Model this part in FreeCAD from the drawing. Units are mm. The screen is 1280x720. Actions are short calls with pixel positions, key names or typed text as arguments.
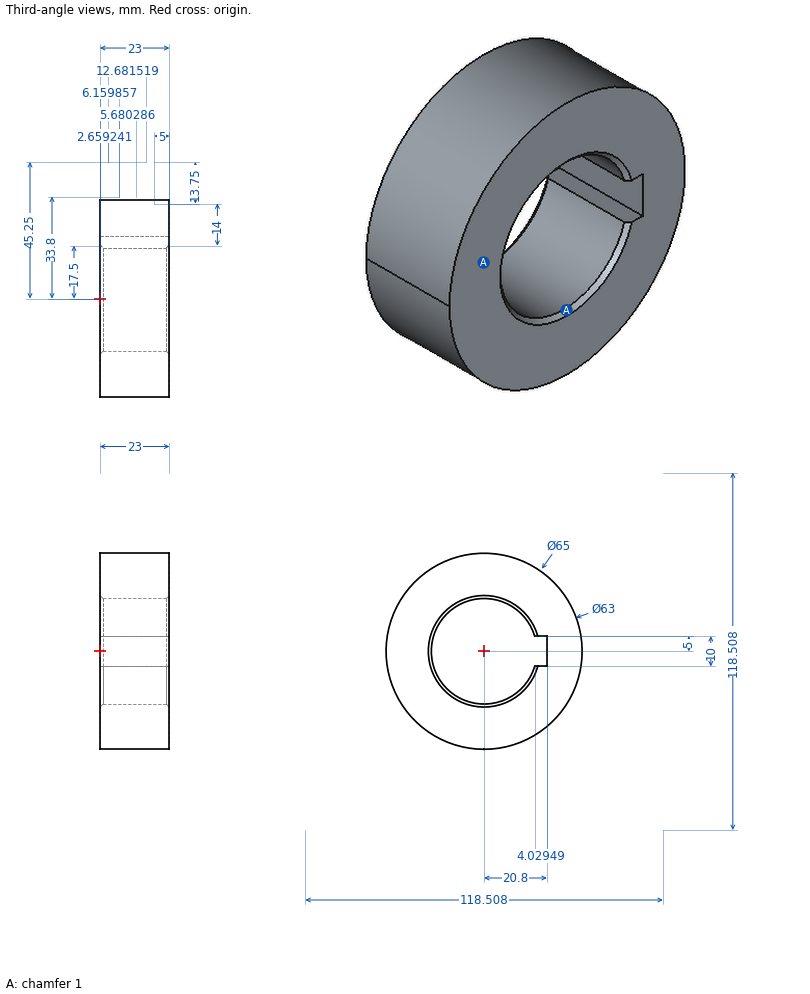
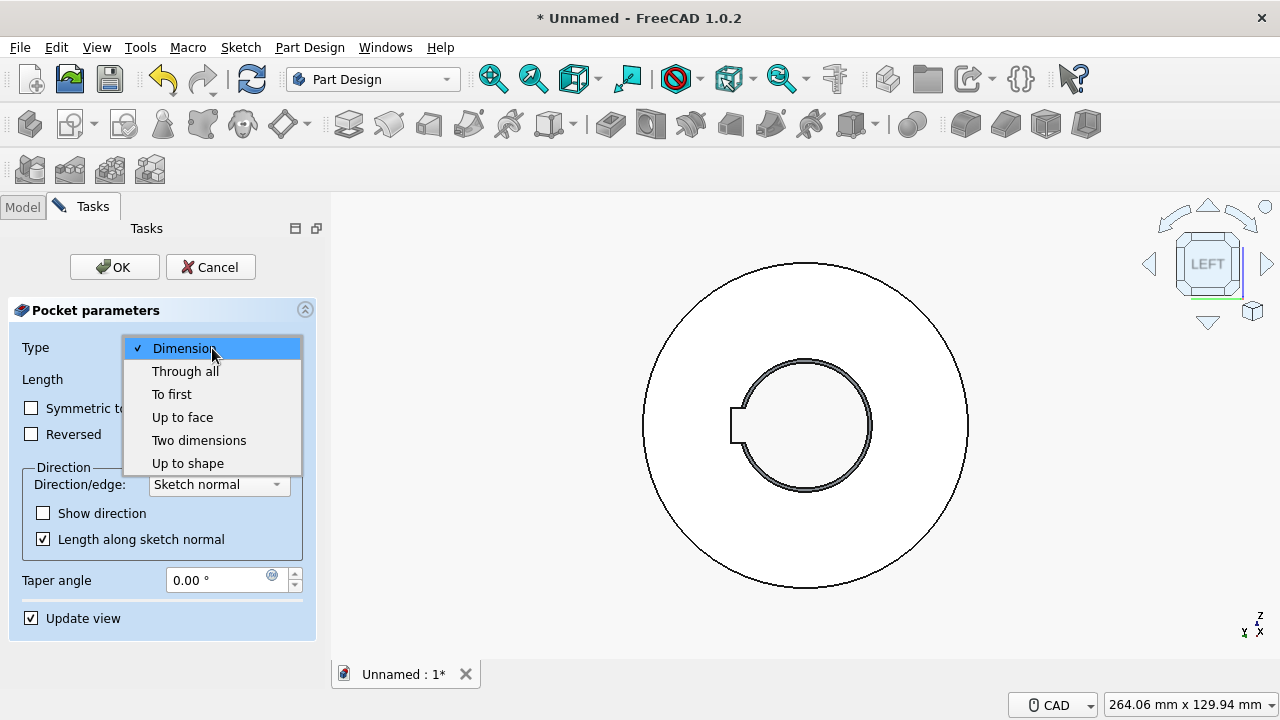
click(212, 440)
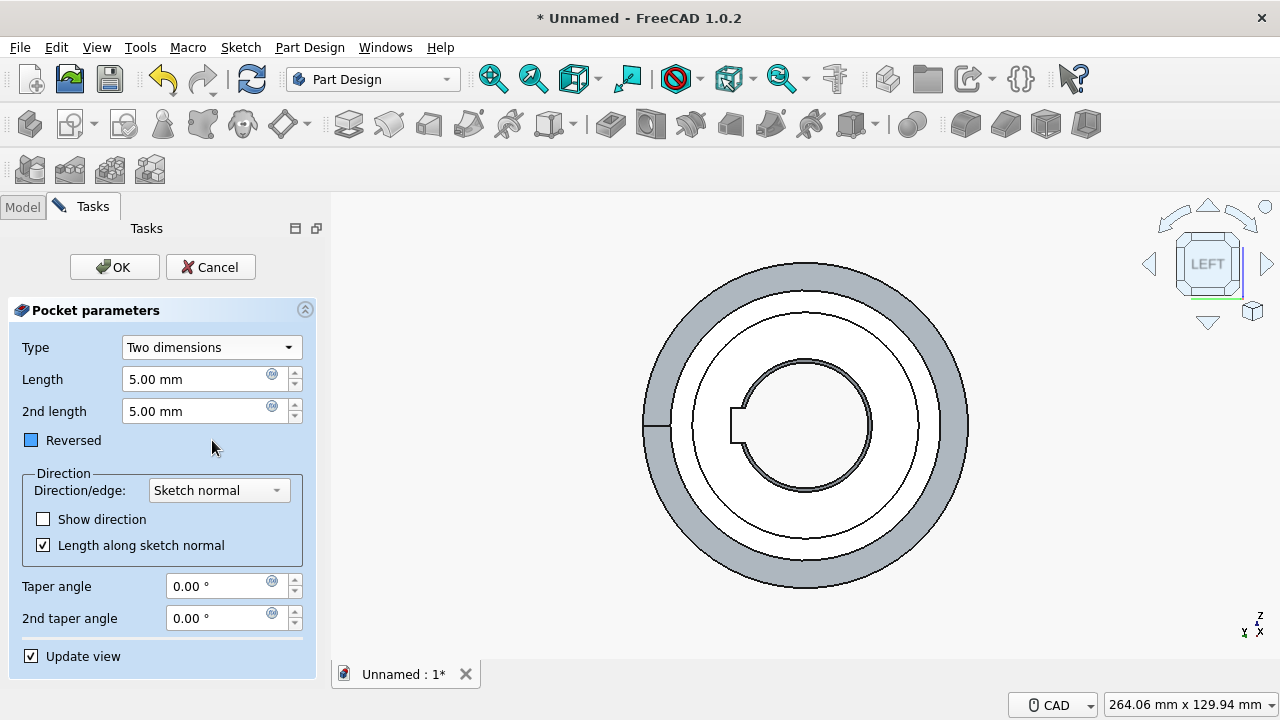
triple_click(204, 379)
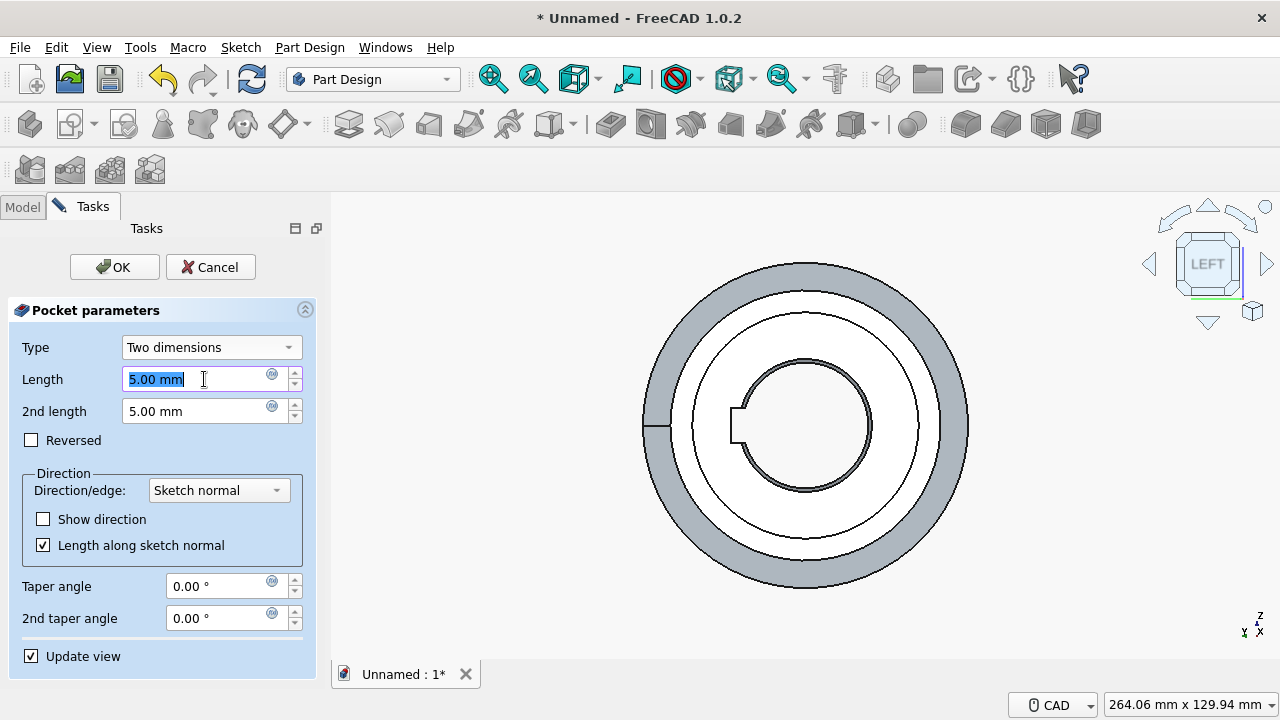
text(23)
key(Tab)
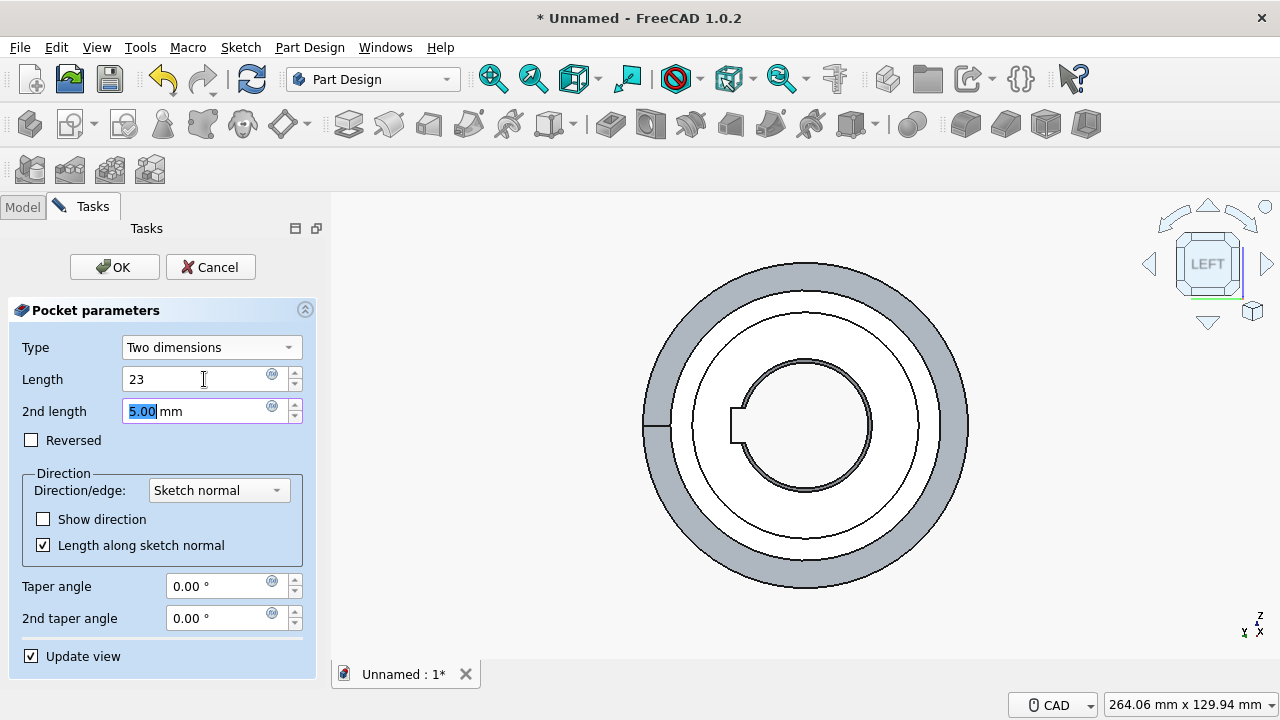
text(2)
key(Tab)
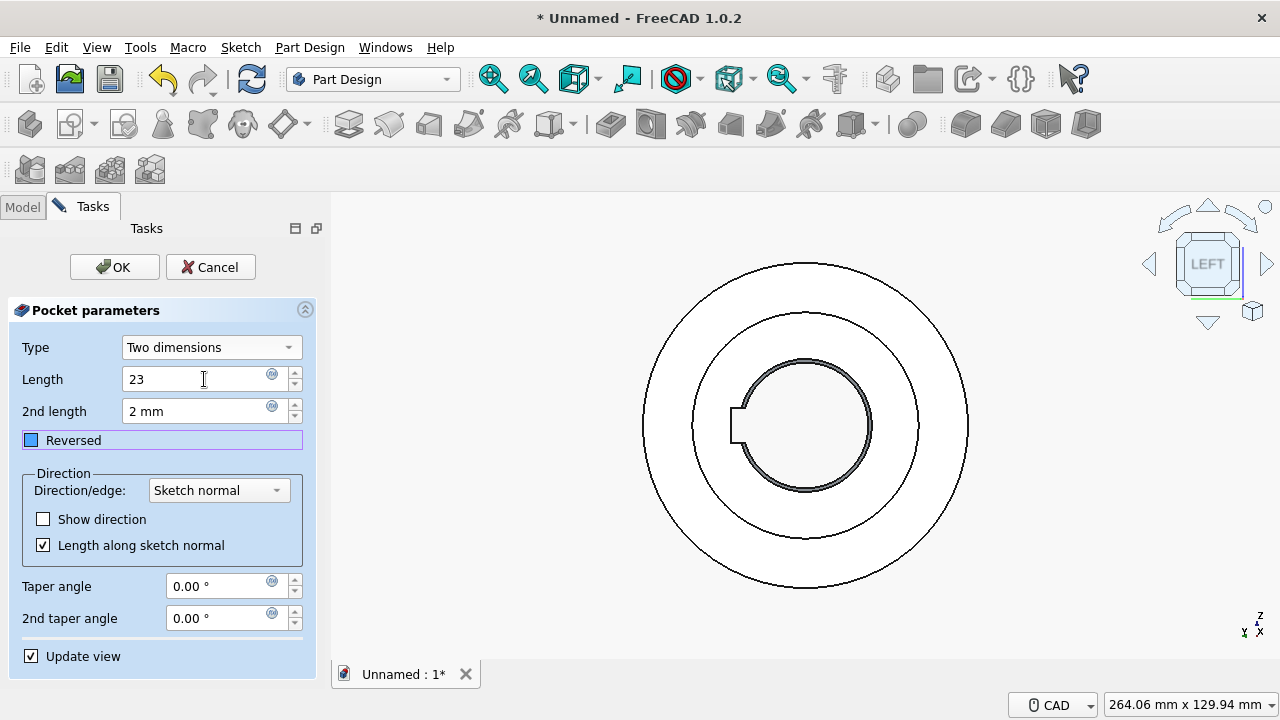
click(30, 440)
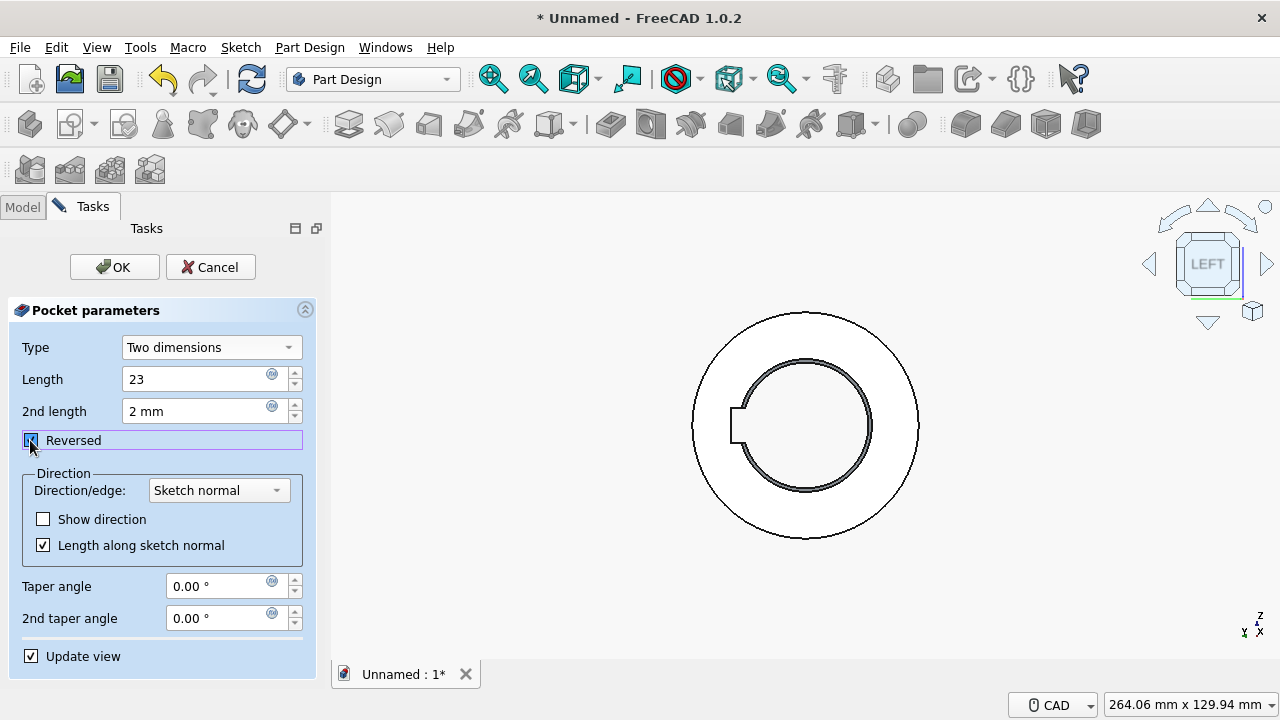
click(115, 267)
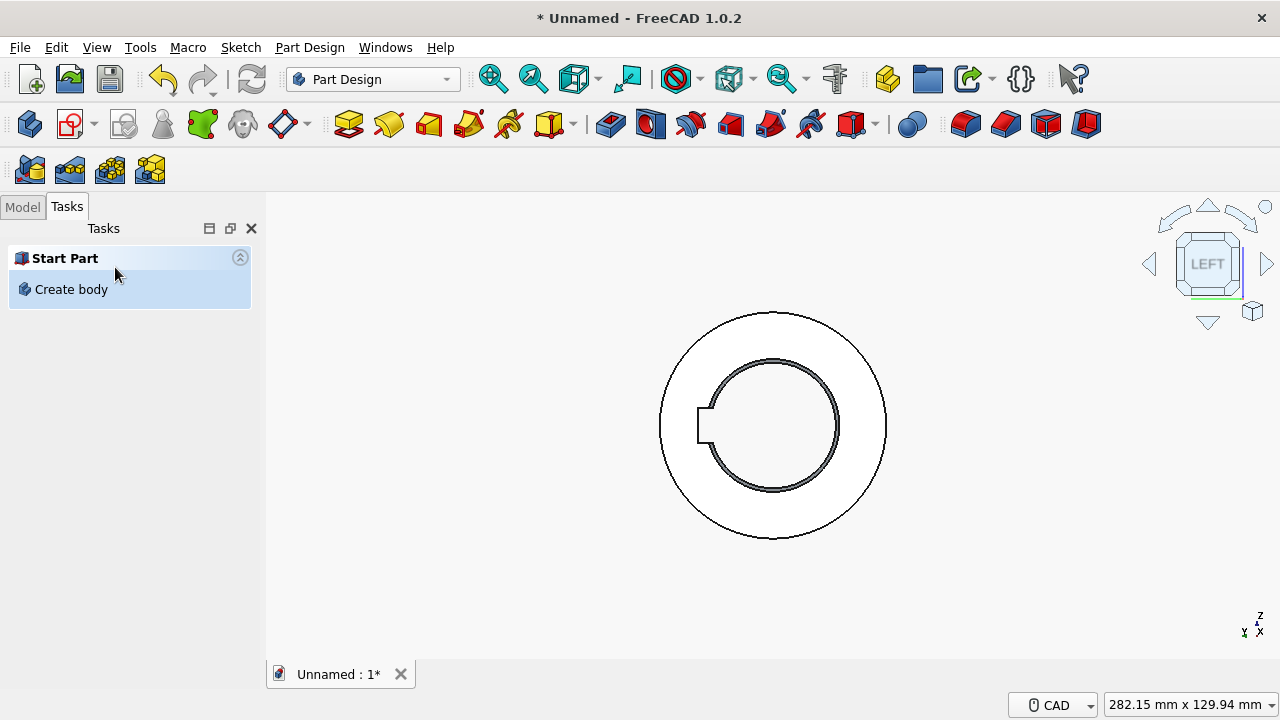
click(838, 489)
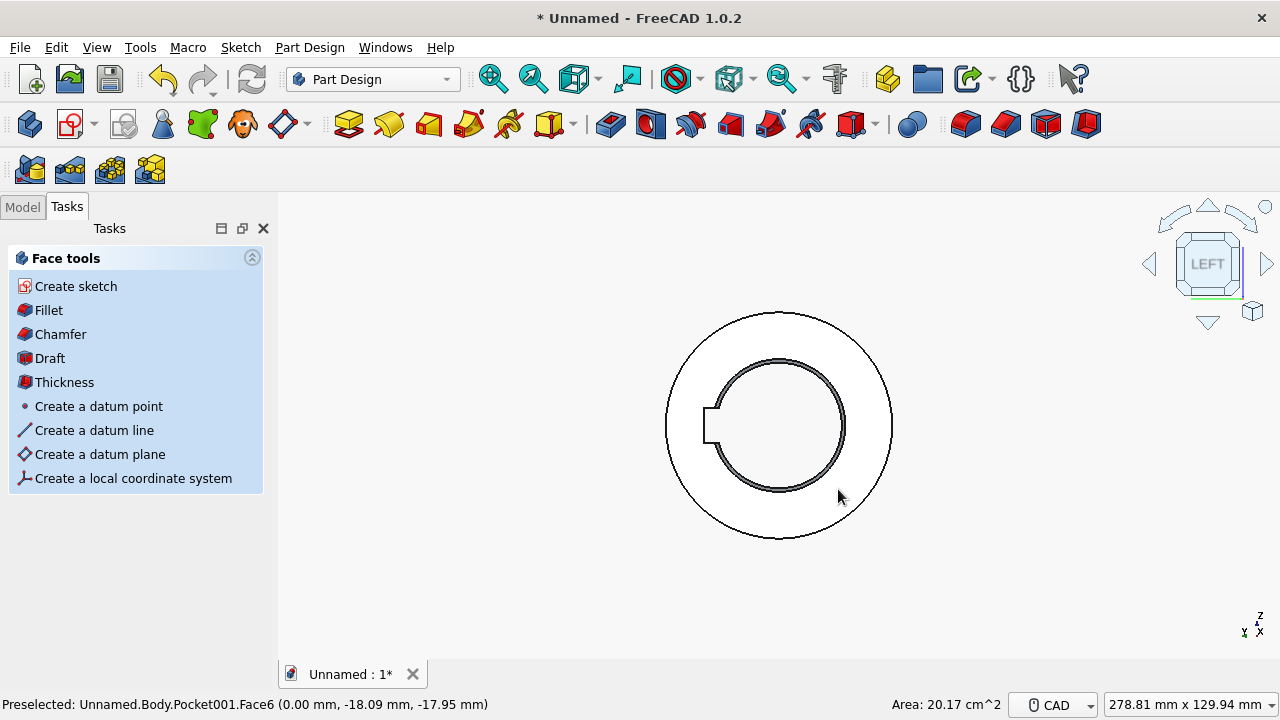
click(70, 124)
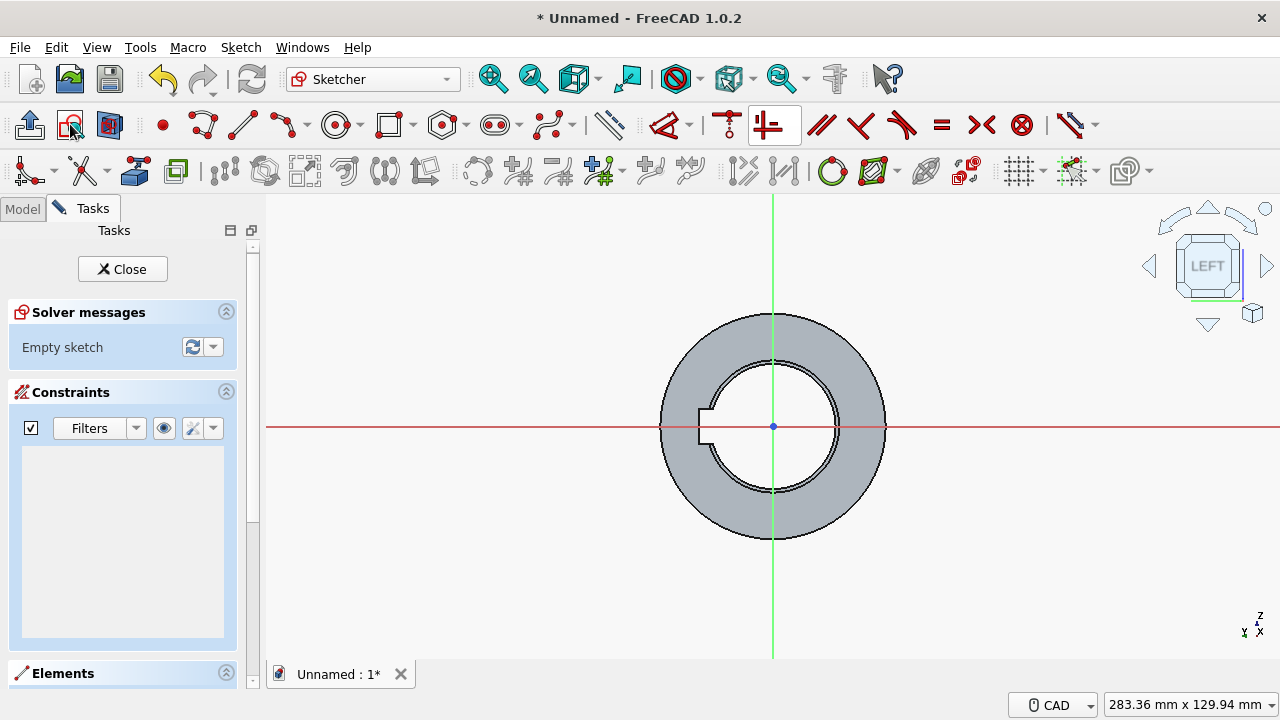
key(g)
key(c)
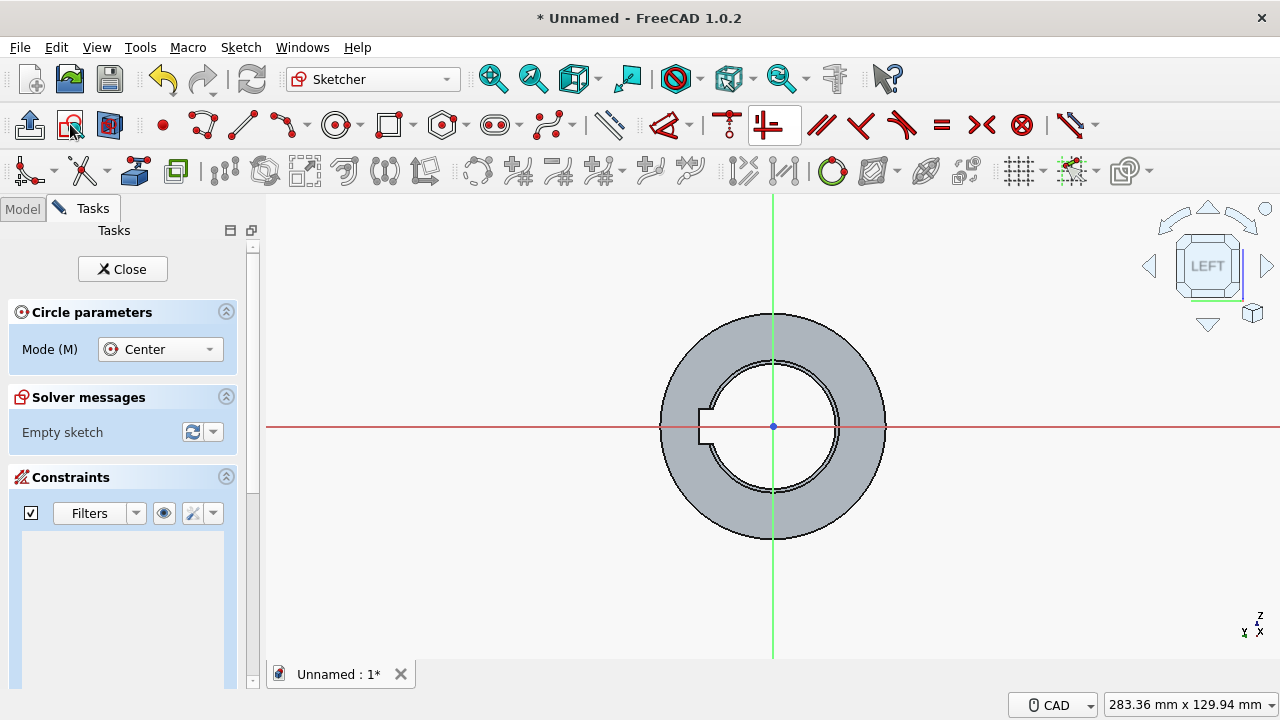
click(773, 427)
move(855, 344)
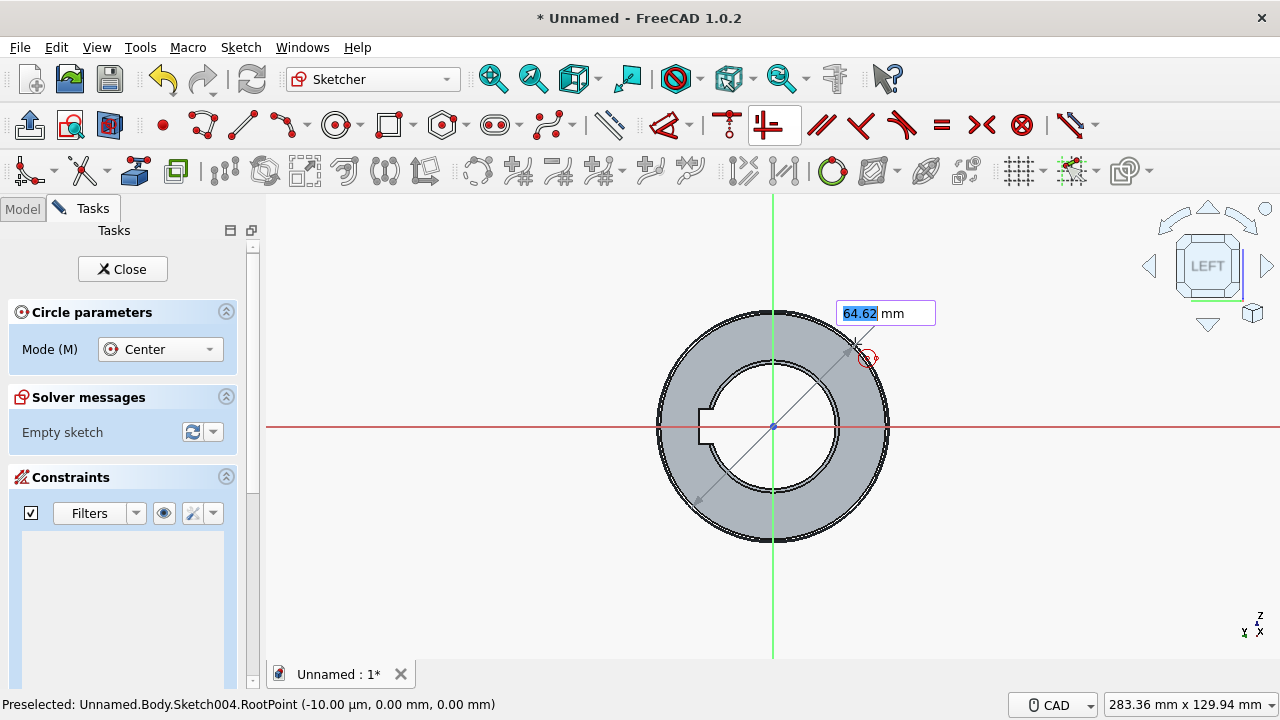
text(65)
key(Return)